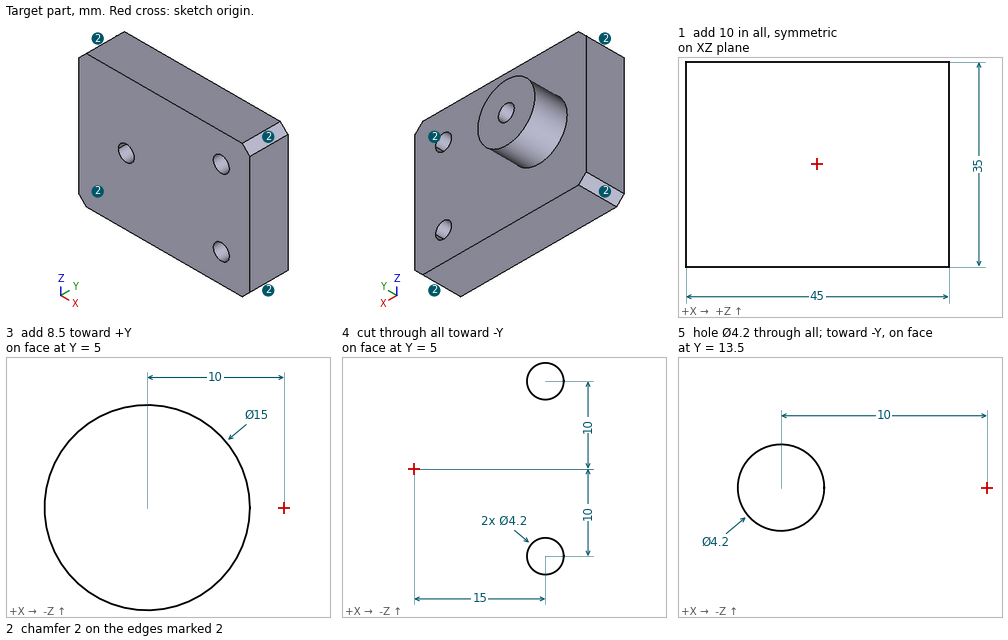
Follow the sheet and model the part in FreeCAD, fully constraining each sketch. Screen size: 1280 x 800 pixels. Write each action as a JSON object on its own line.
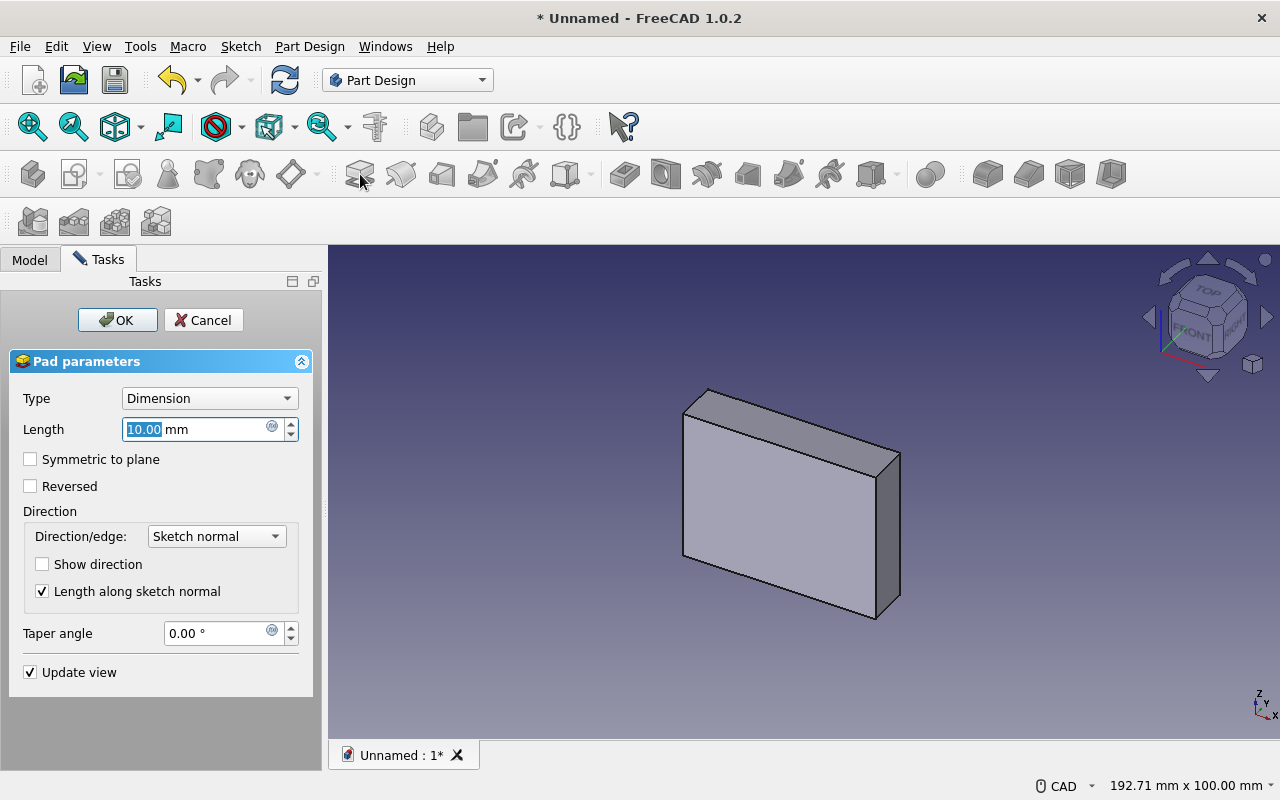
{"action": "type", "text": "10"}
{"action": "key", "text": "Tab"}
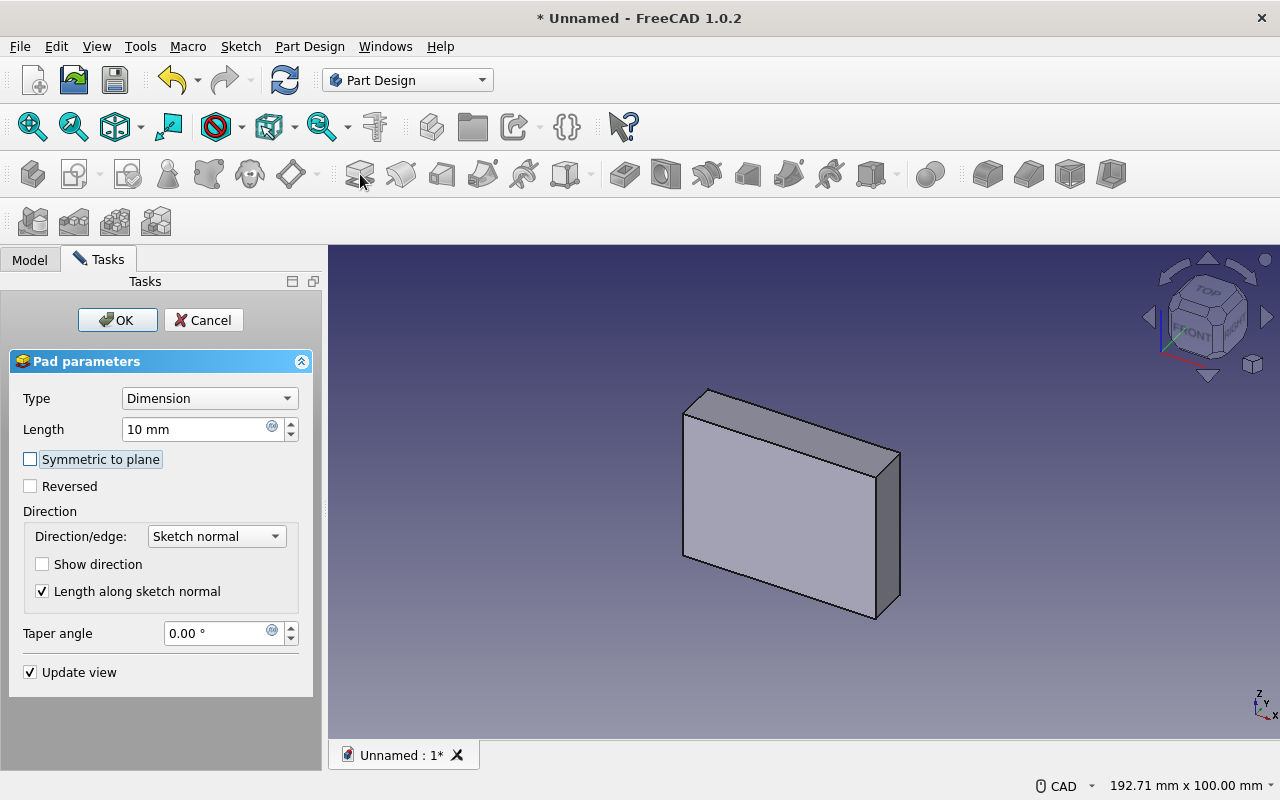
{"action": "left_click", "coordinate": [31, 459]}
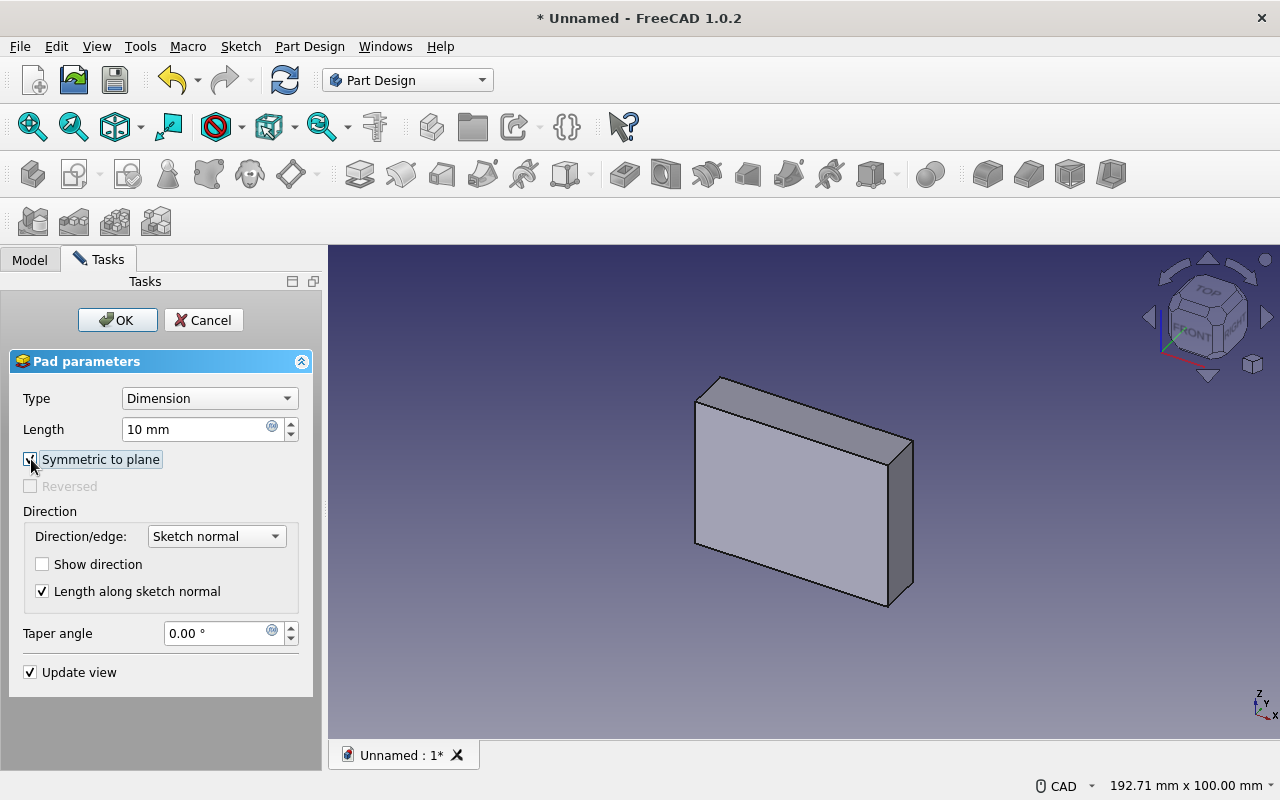
{"action": "left_click", "coordinate": [118, 320]}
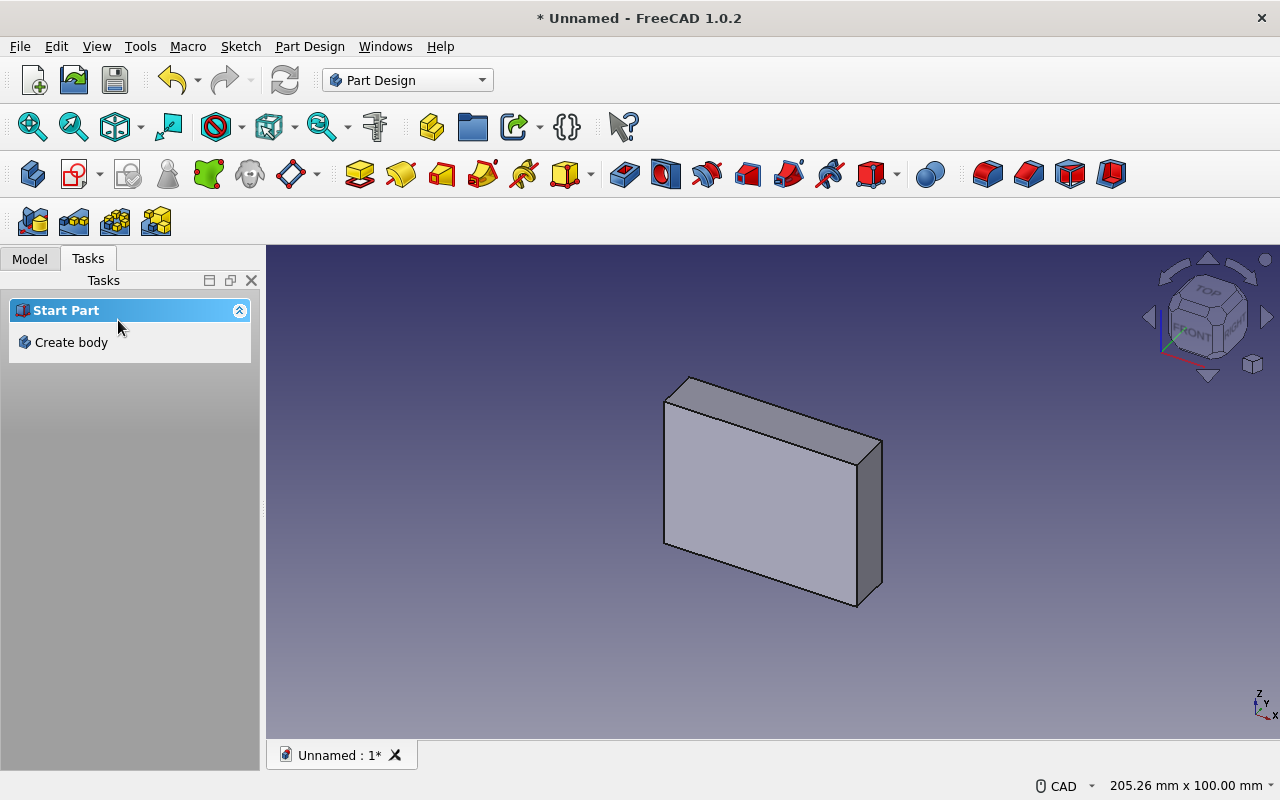
{"action": "left_click", "coordinate": [869, 452]}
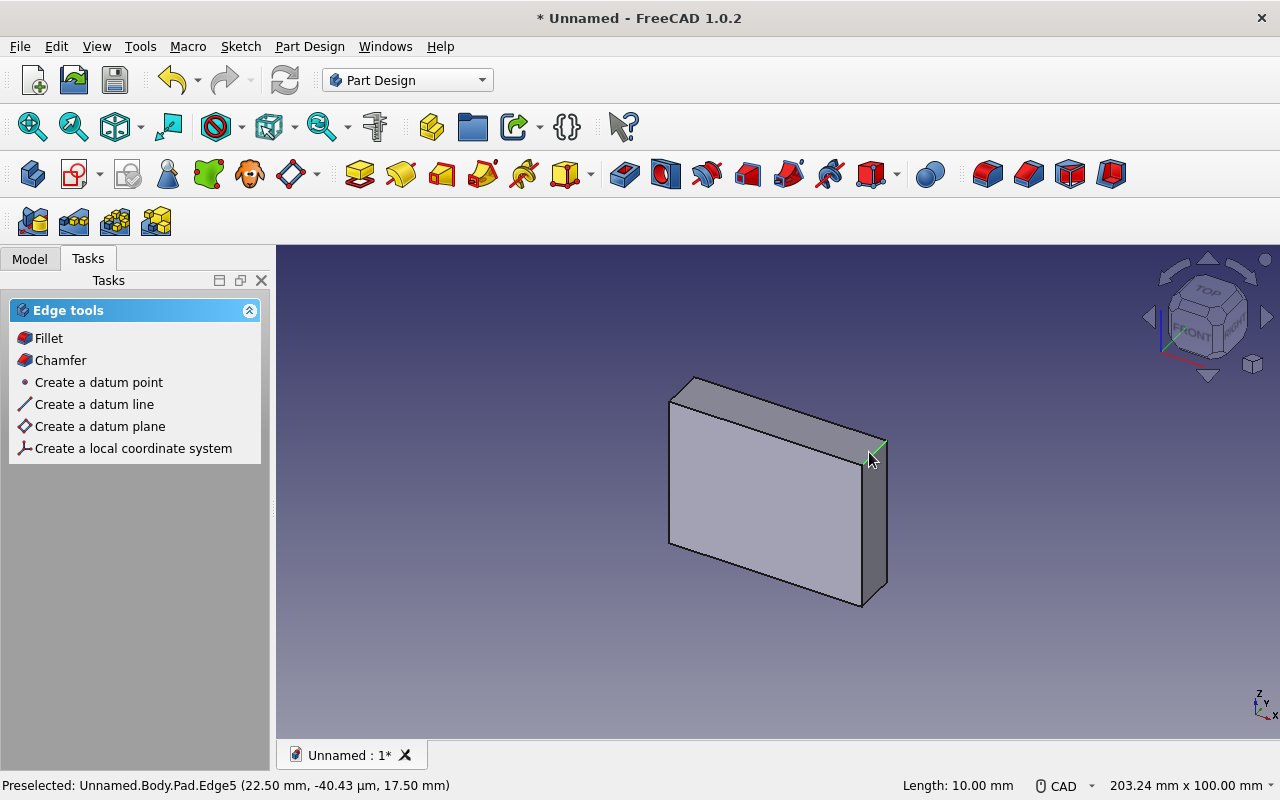
{"action": "key", "text": "0"}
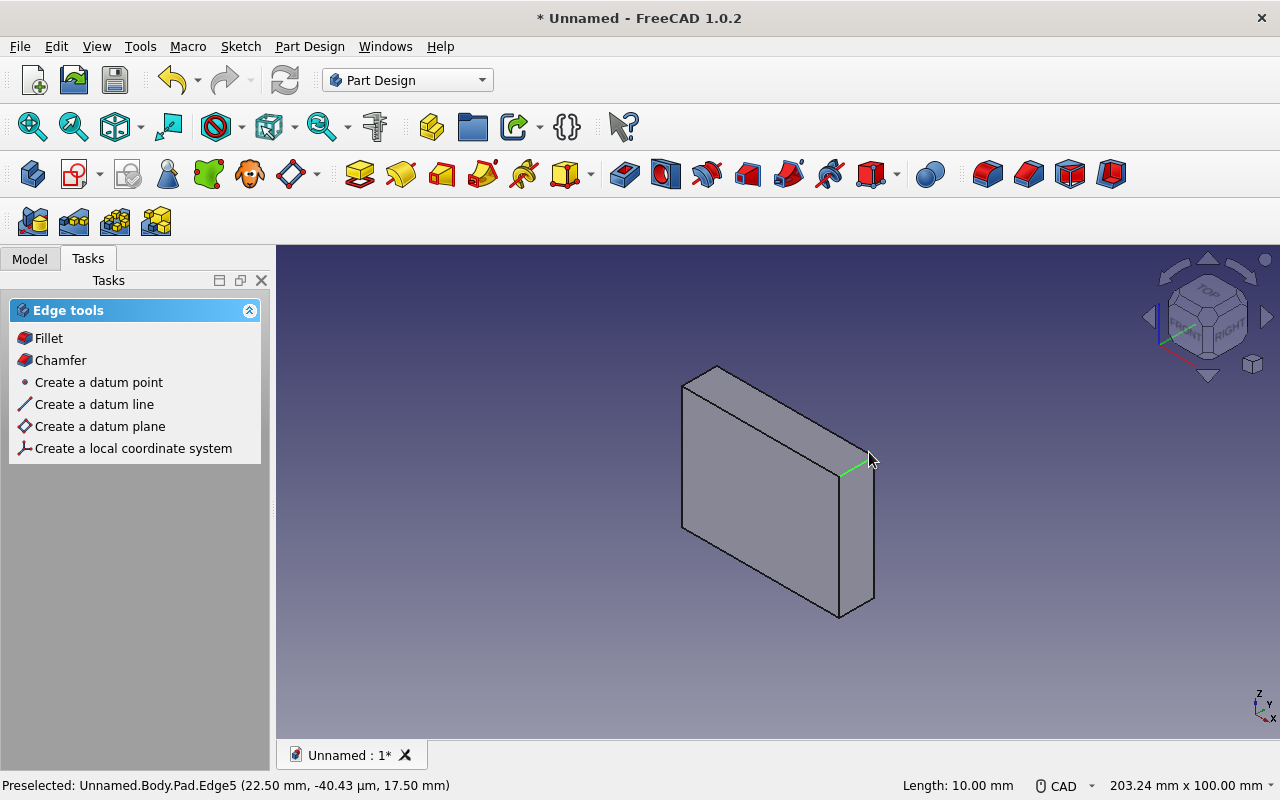
{"action": "key", "text": "2"}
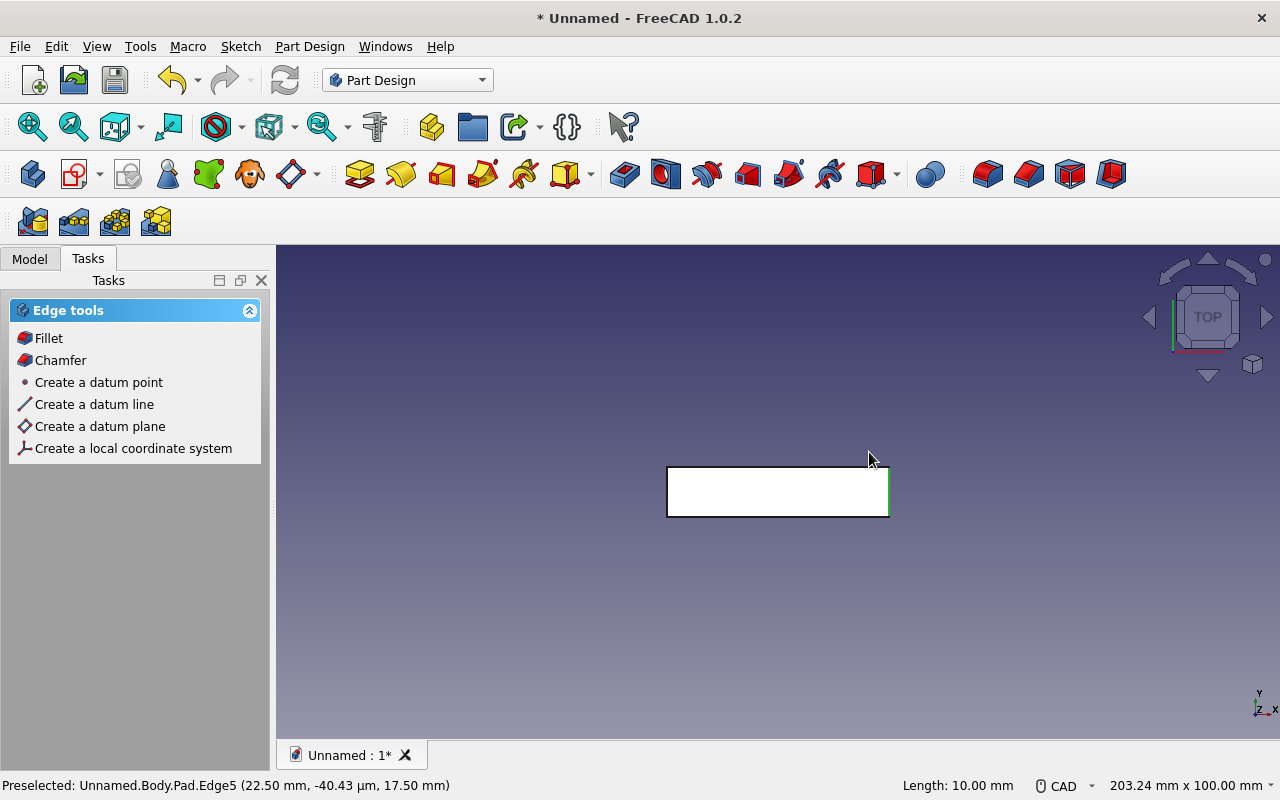
{"action": "key", "text": "v f"}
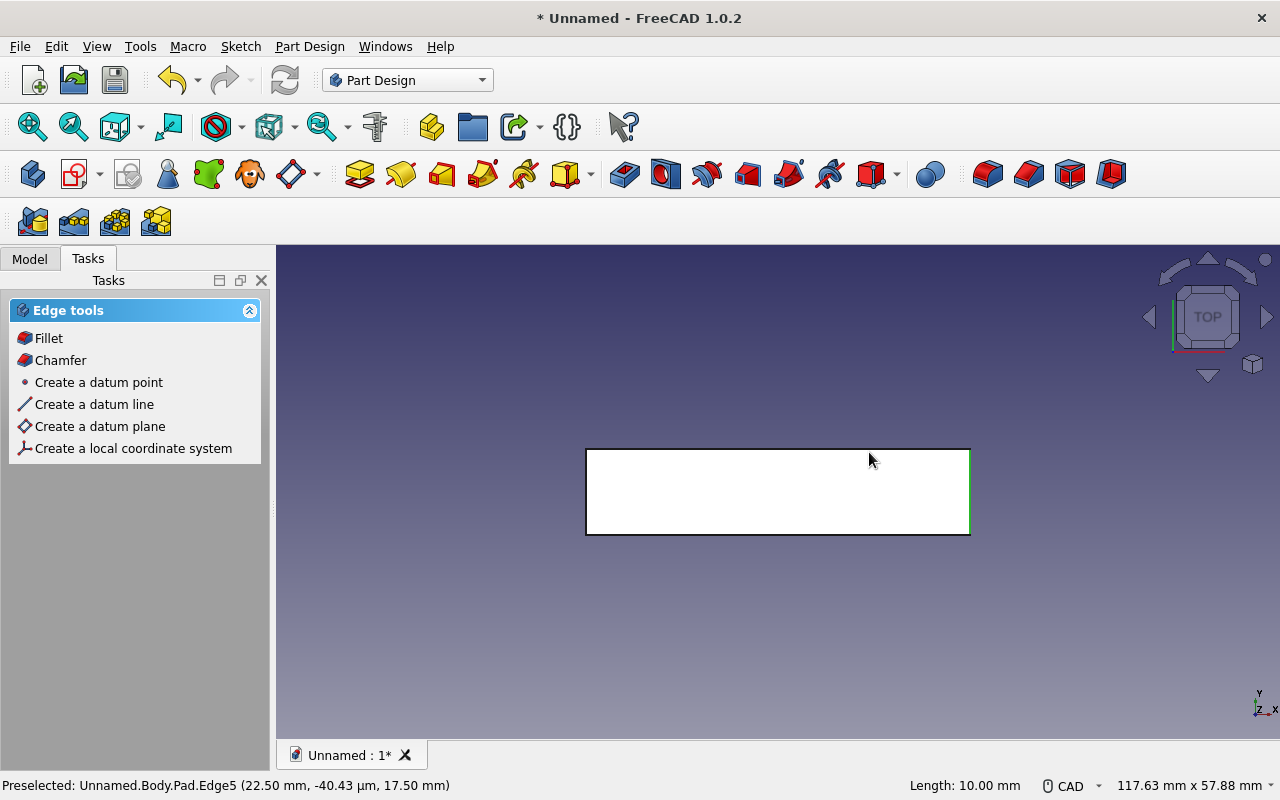
{"action": "left_click", "coordinate": [586, 491], "text": "ctrl"}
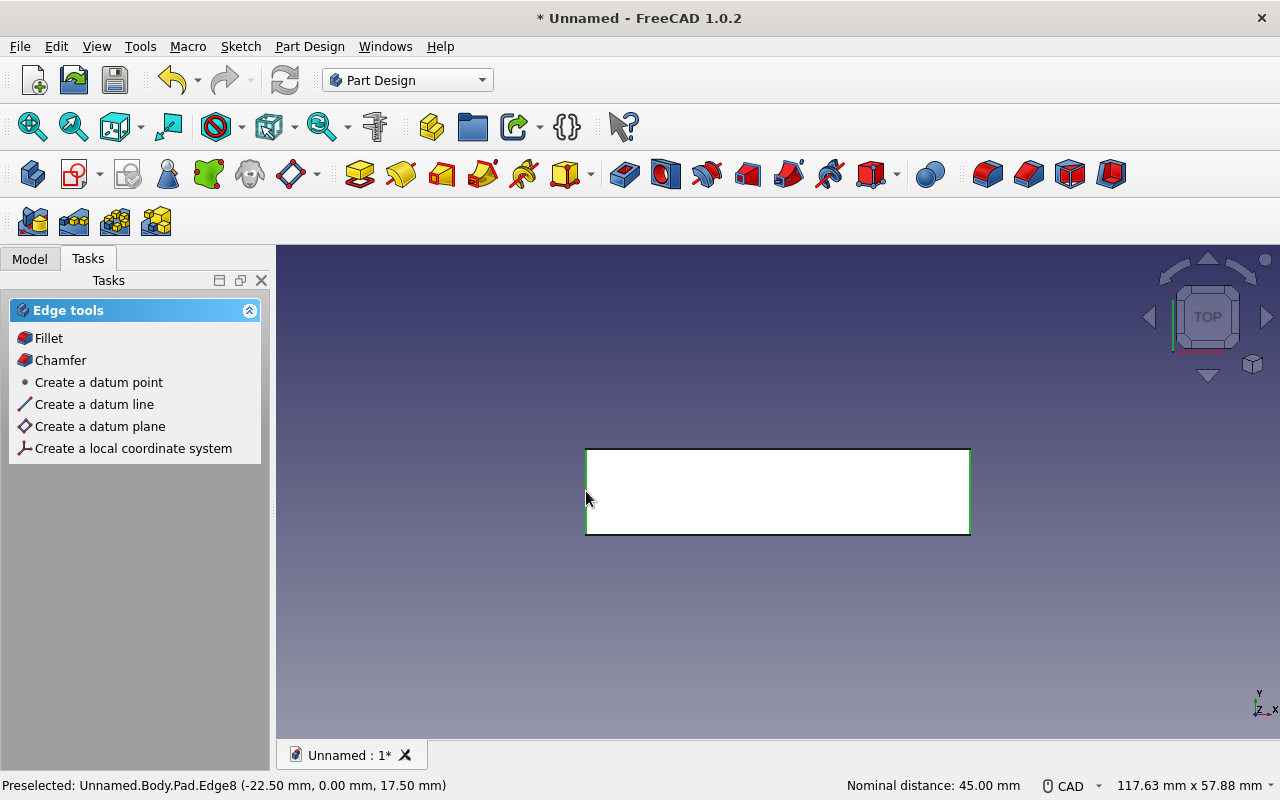
{"action": "key", "text": "1"}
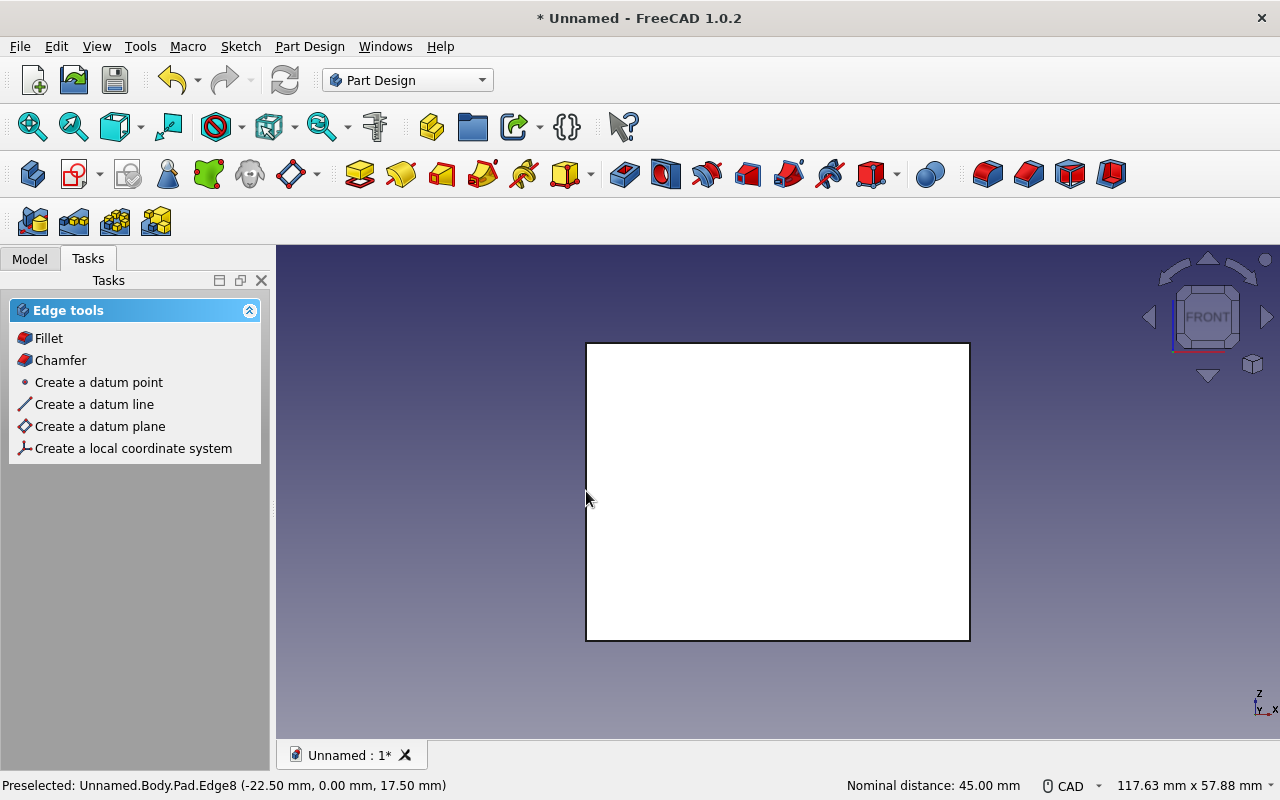
{"action": "key", "text": "3"}